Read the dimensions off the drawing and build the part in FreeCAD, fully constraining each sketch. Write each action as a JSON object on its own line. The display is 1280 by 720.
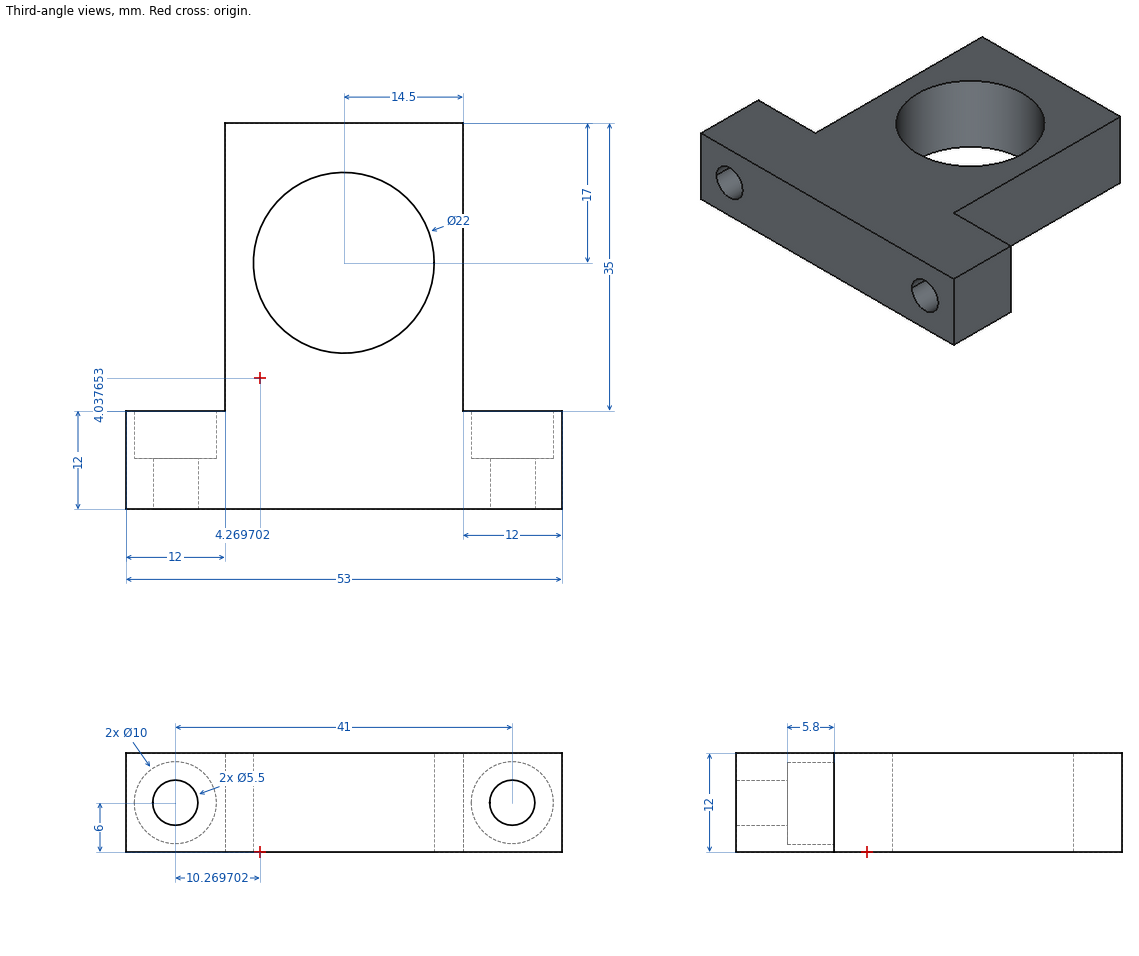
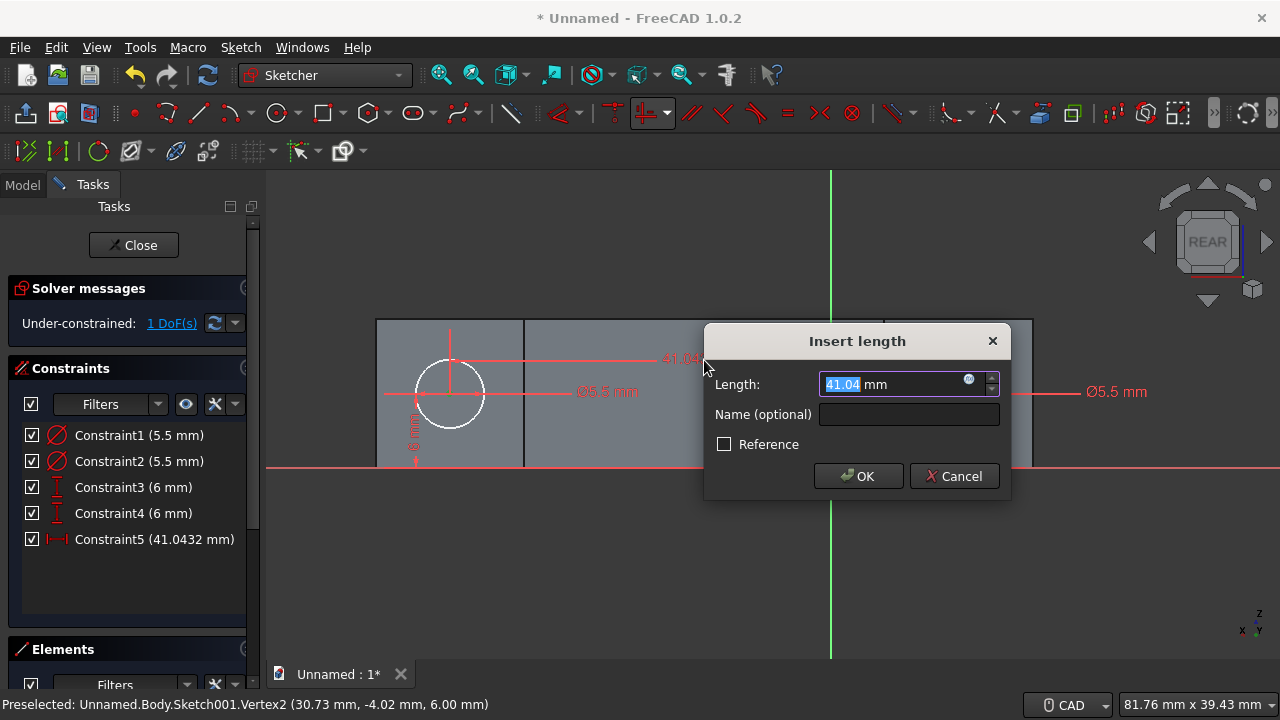
{"action": "type", "text": "41"}
{"action": "key", "text": "Return"}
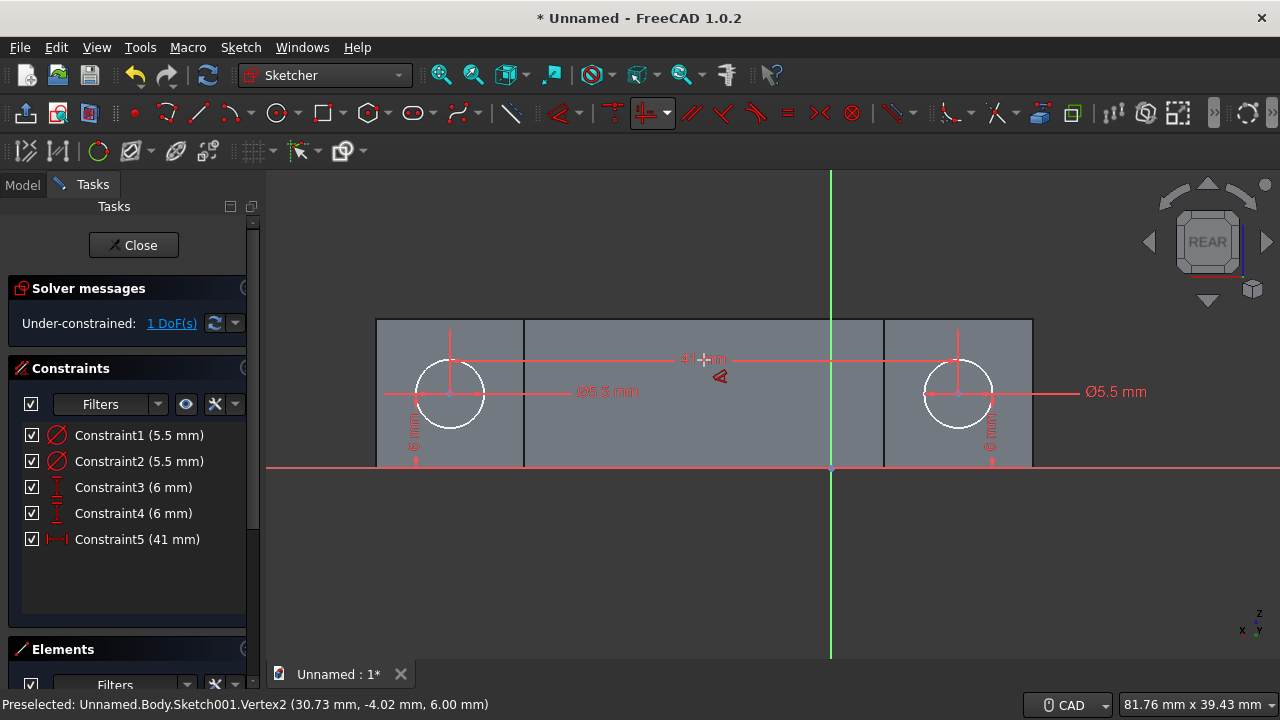
{"action": "left_click", "coordinate": [958, 394]}
{"action": "left_click", "coordinate": [895, 502]}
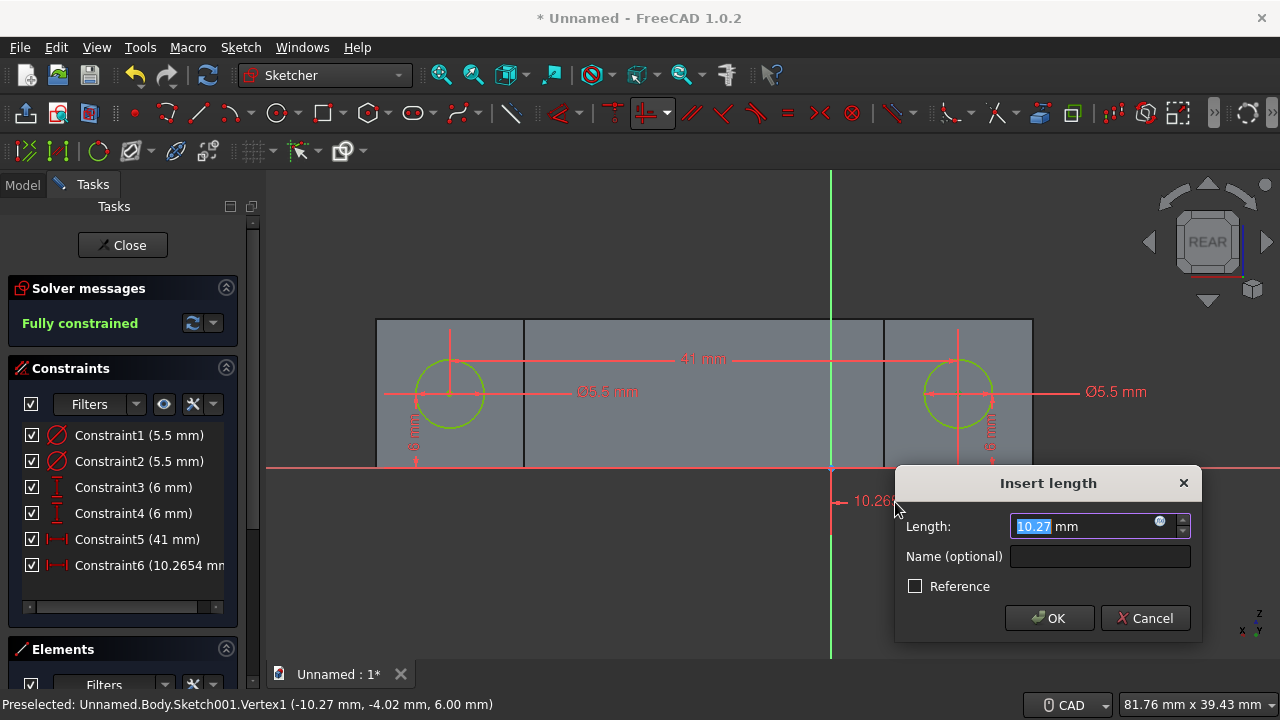
{"action": "type", "text": "10.269702"}
{"action": "key", "text": "Return"}
{"action": "key", "text": "Escape"}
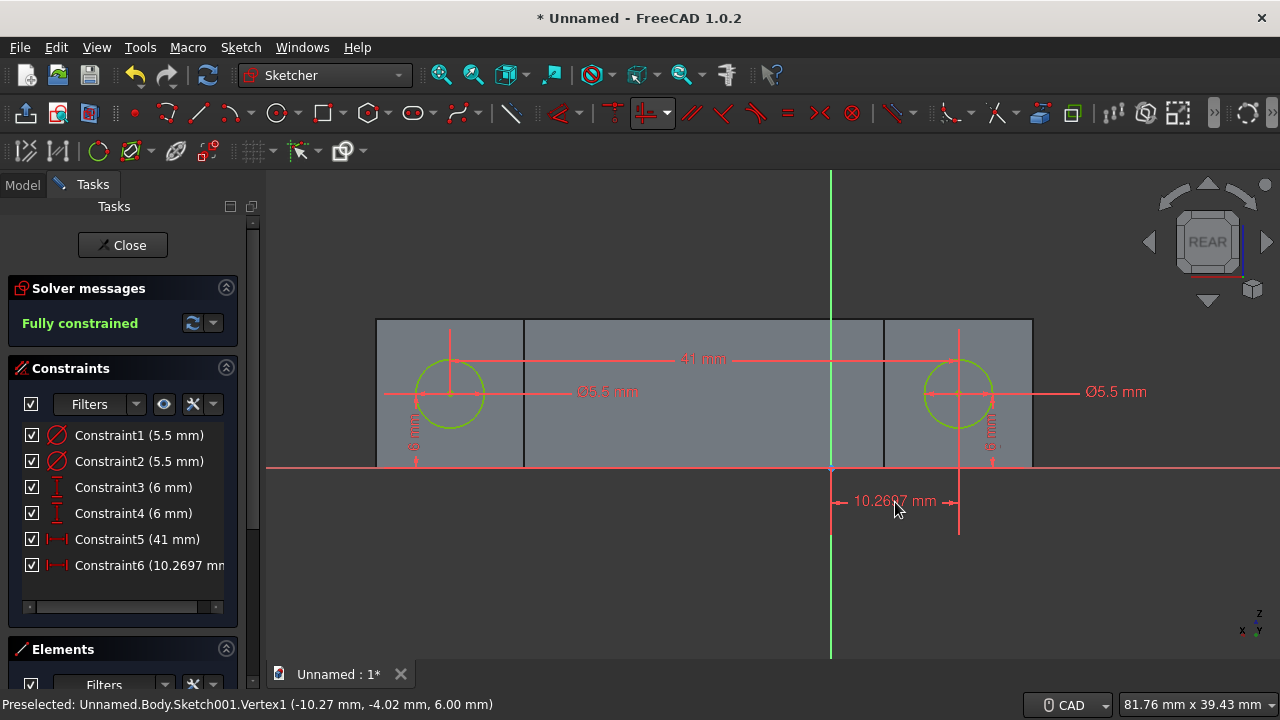
{"action": "left_click", "coordinate": [123, 245]}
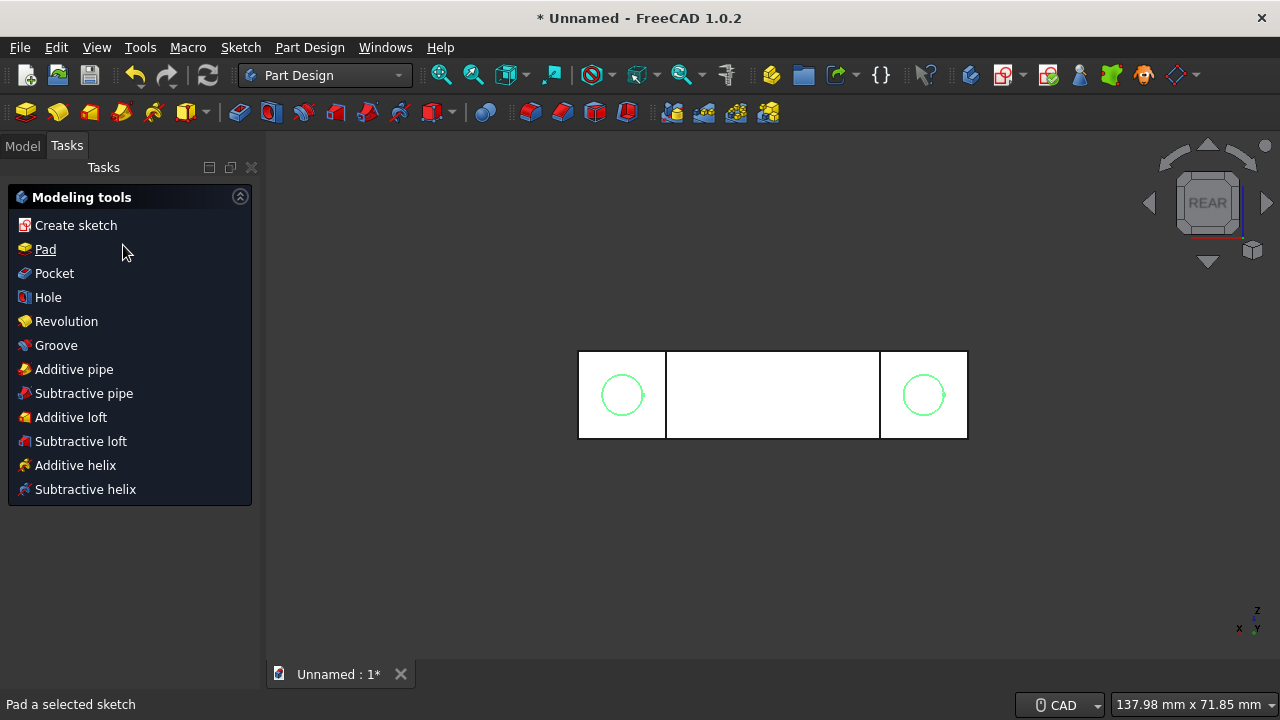
{"action": "left_click", "coordinate": [240, 112]}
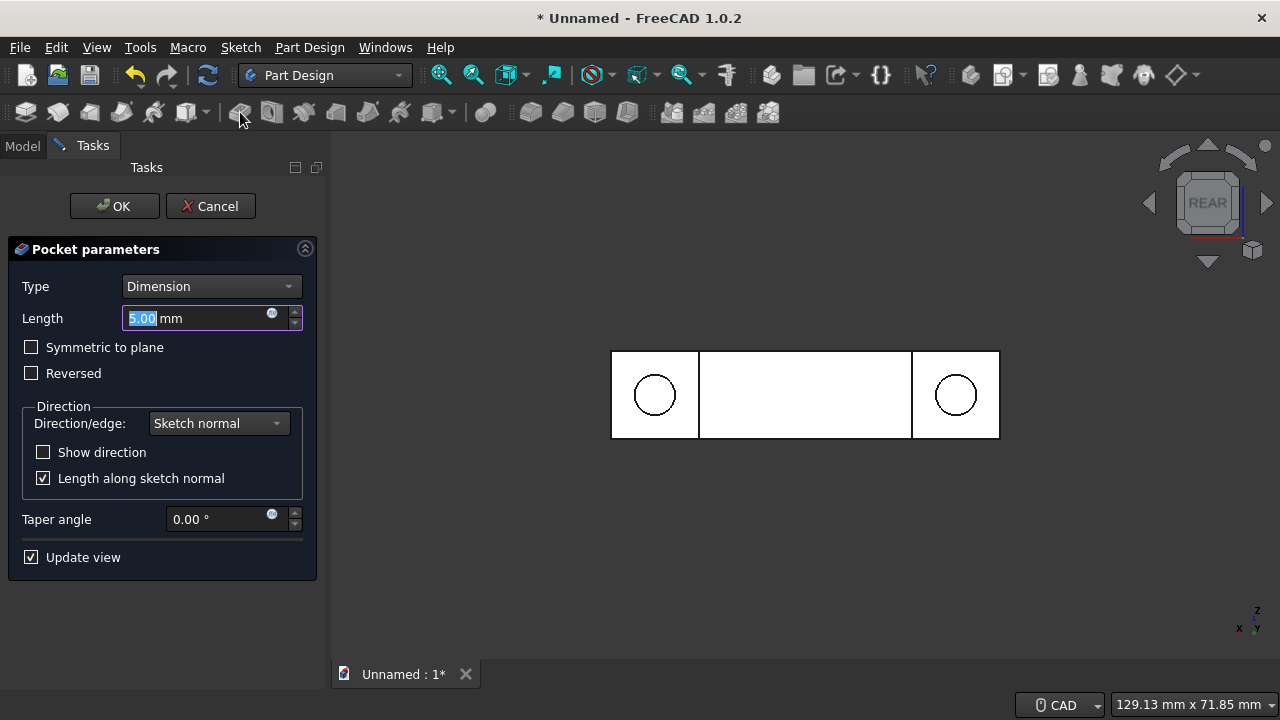
{"action": "left_click", "coordinate": [212, 286]}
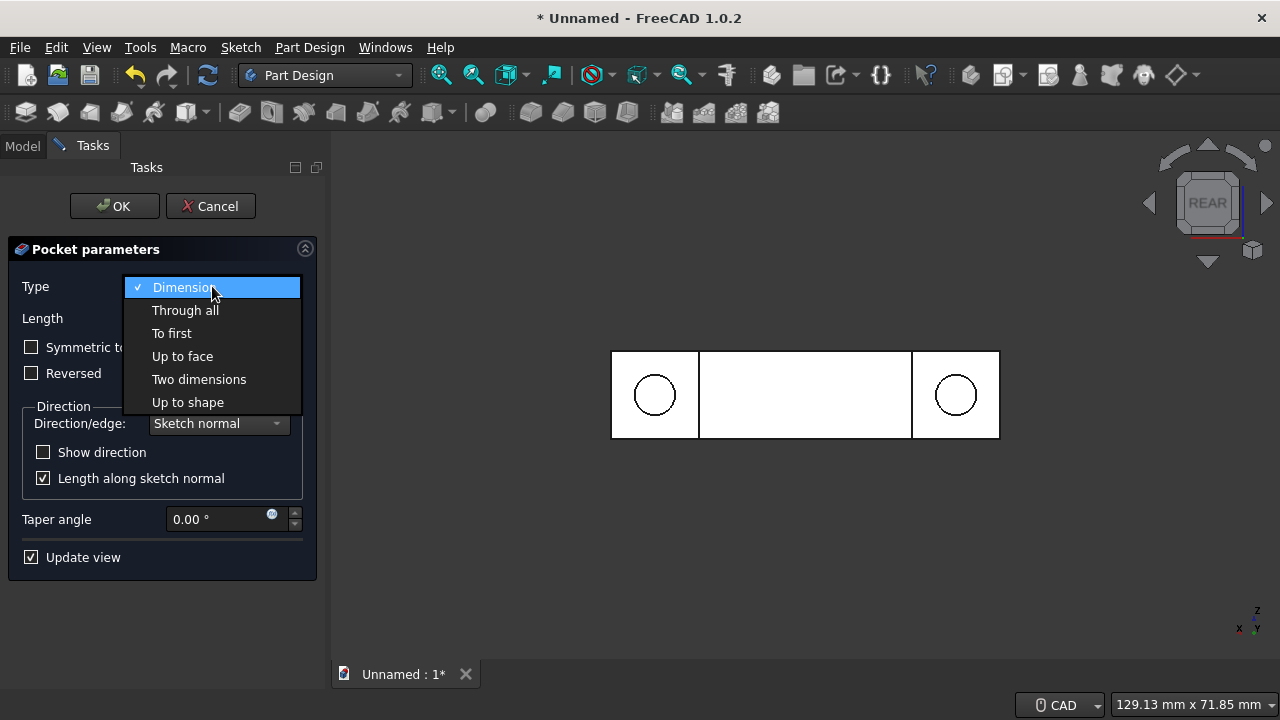
{"action": "left_click", "coordinate": [212, 310]}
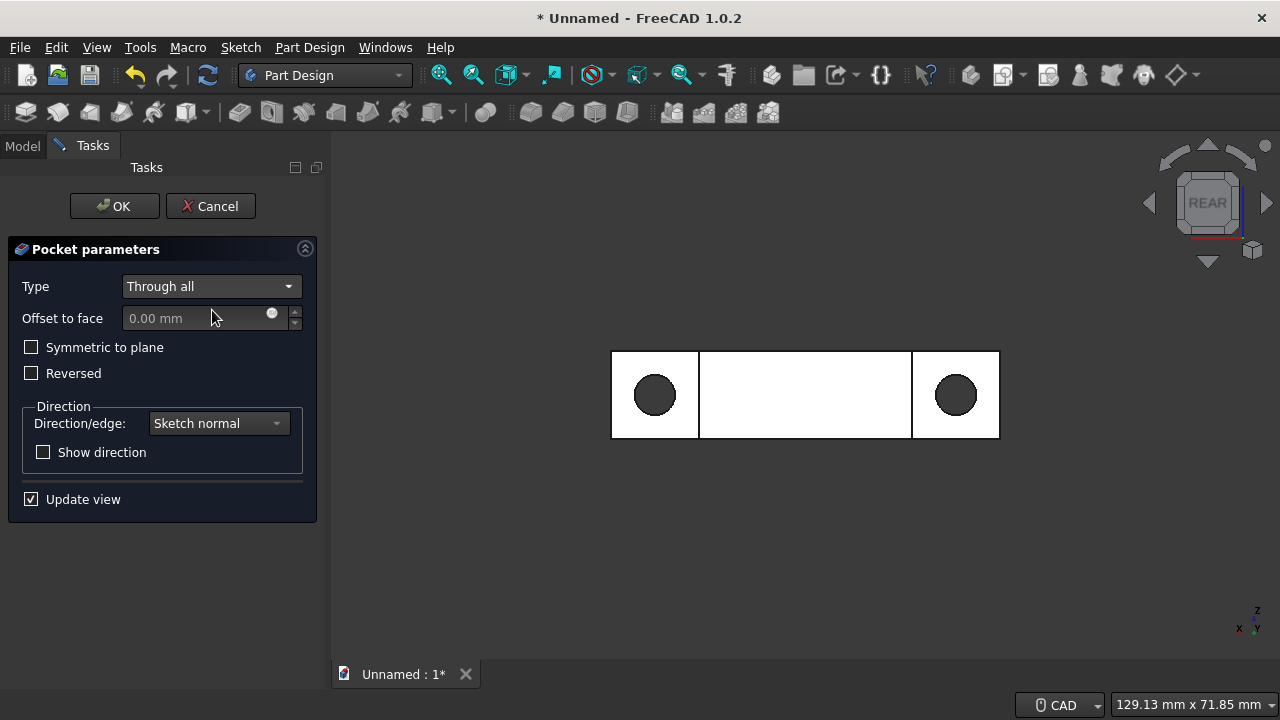
{"action": "left_click", "coordinate": [115, 206]}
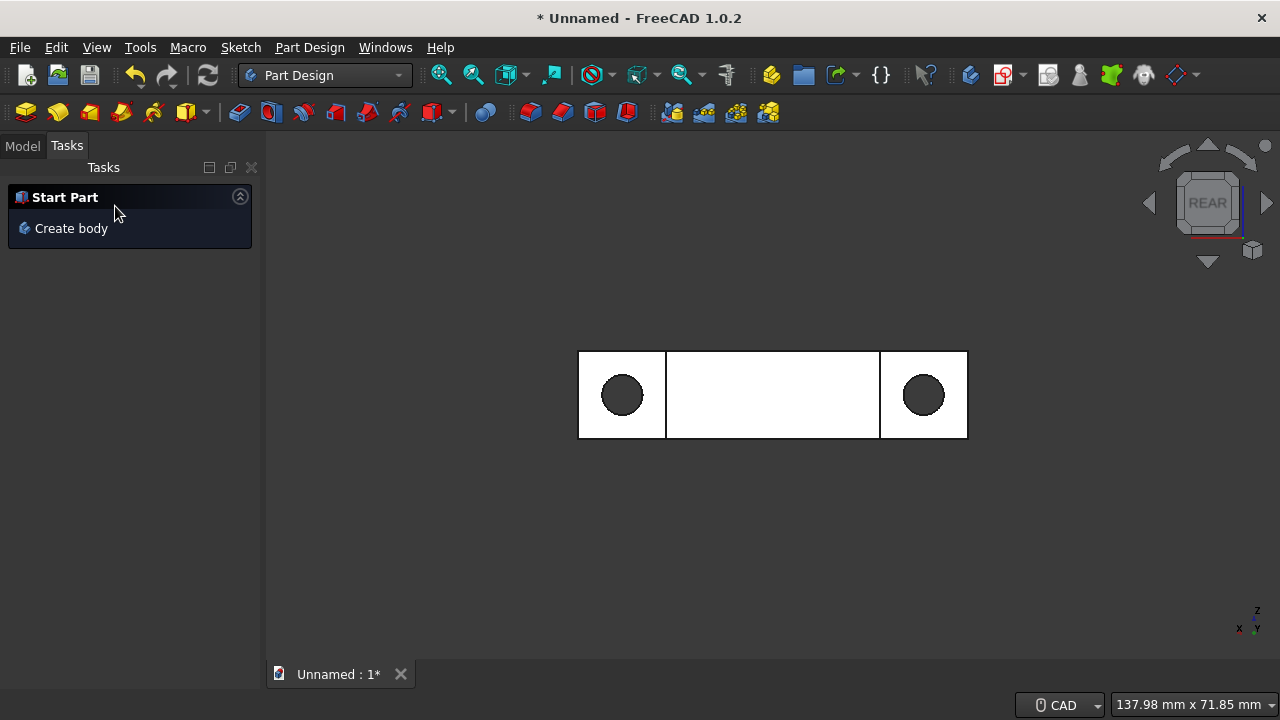
{"action": "left_click", "coordinate": [442, 76]}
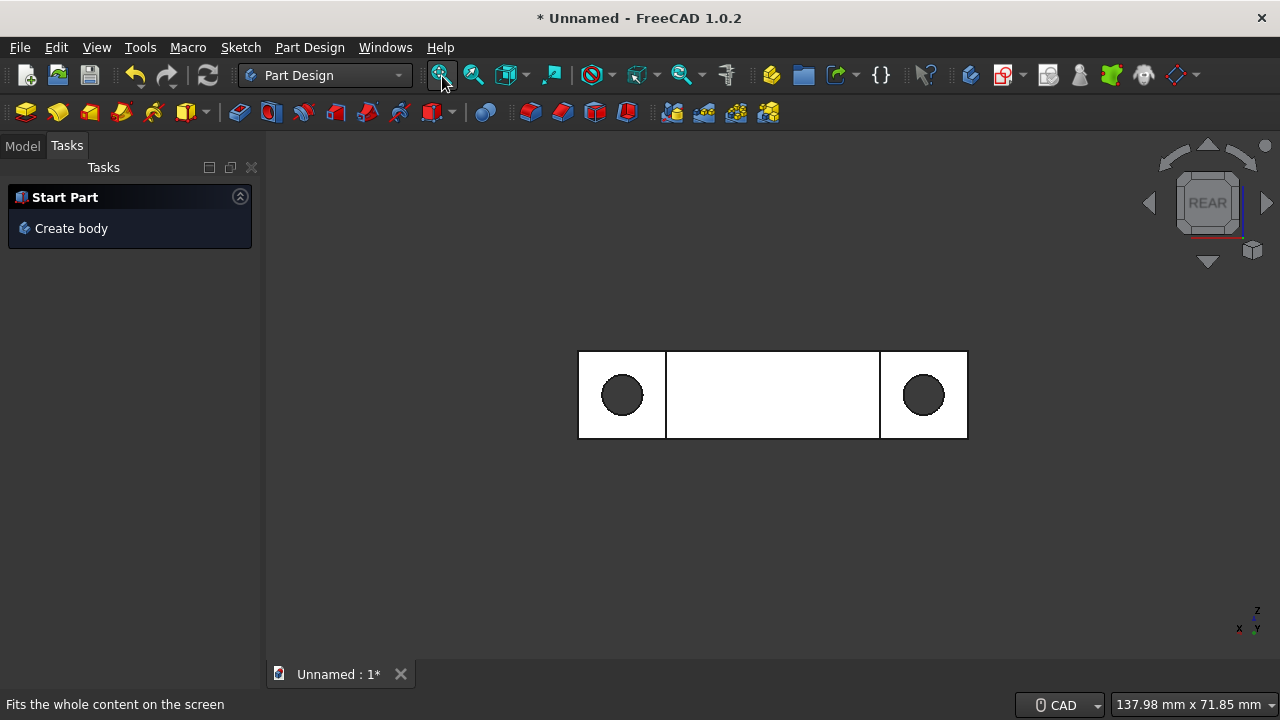
{"action": "left_click", "coordinate": [648, 369]}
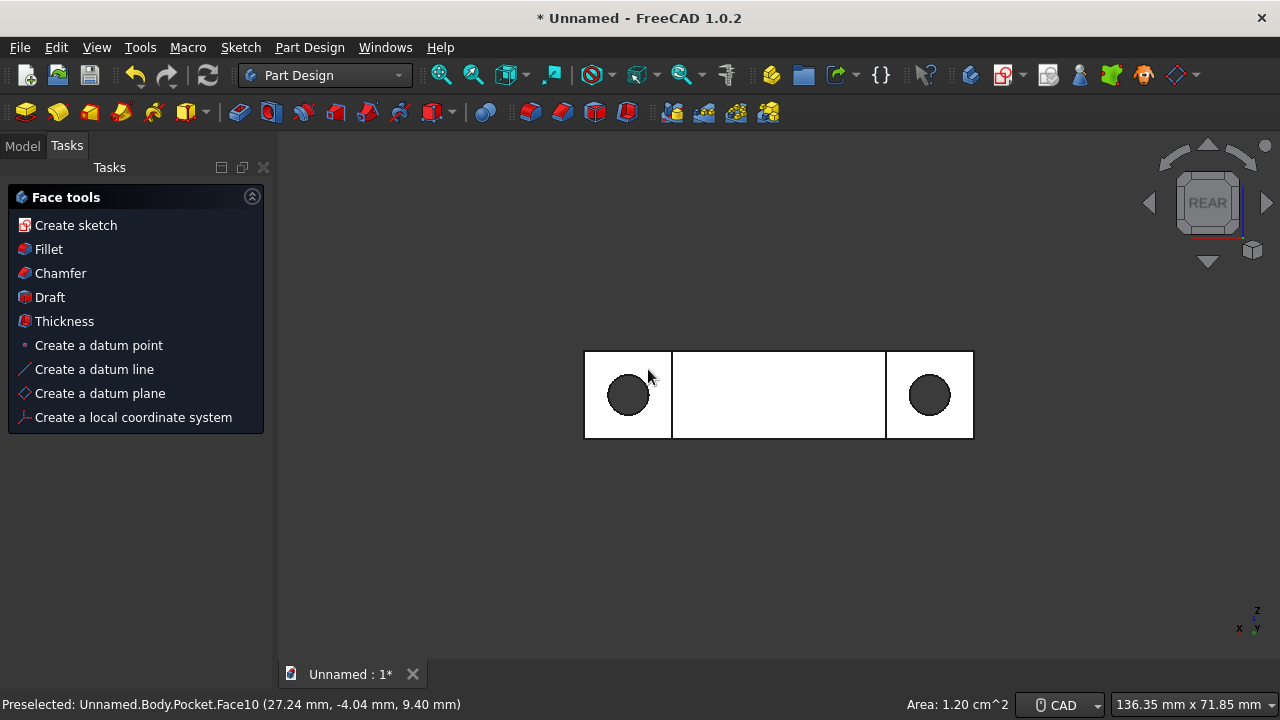
{"action": "left_click", "coordinate": [1004, 76]}